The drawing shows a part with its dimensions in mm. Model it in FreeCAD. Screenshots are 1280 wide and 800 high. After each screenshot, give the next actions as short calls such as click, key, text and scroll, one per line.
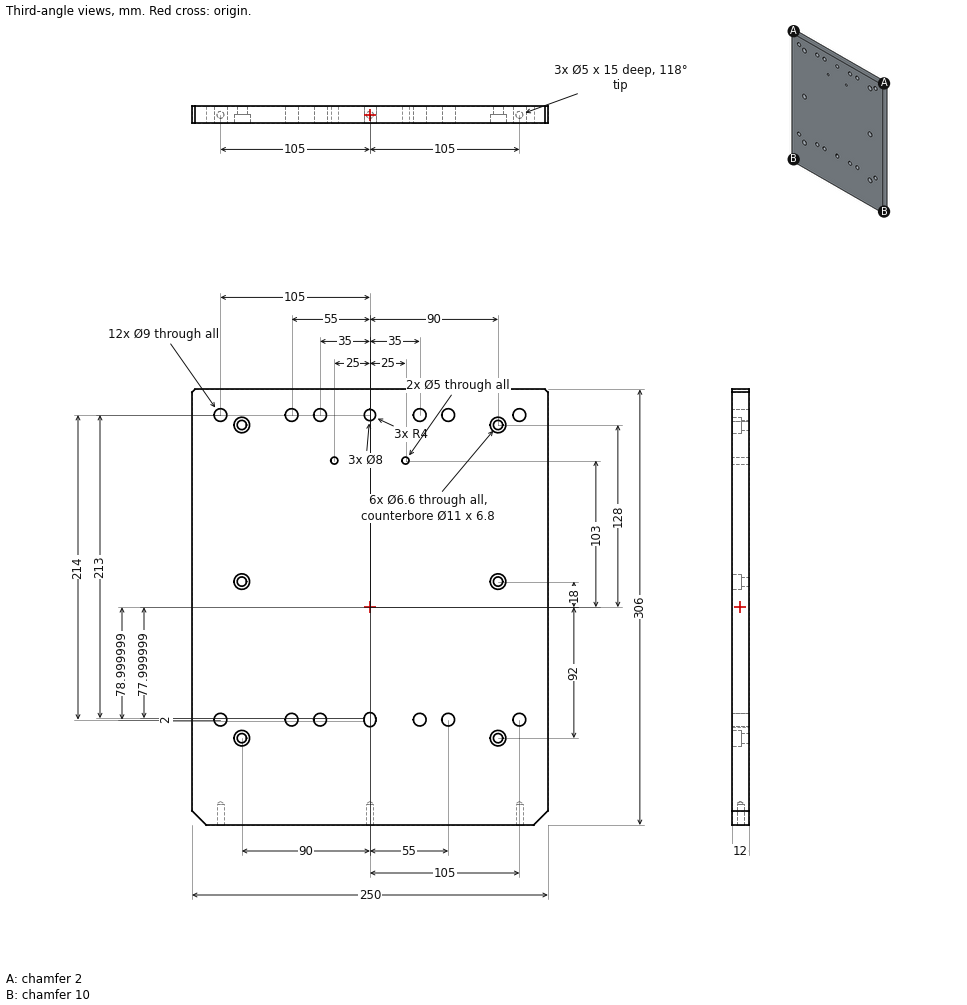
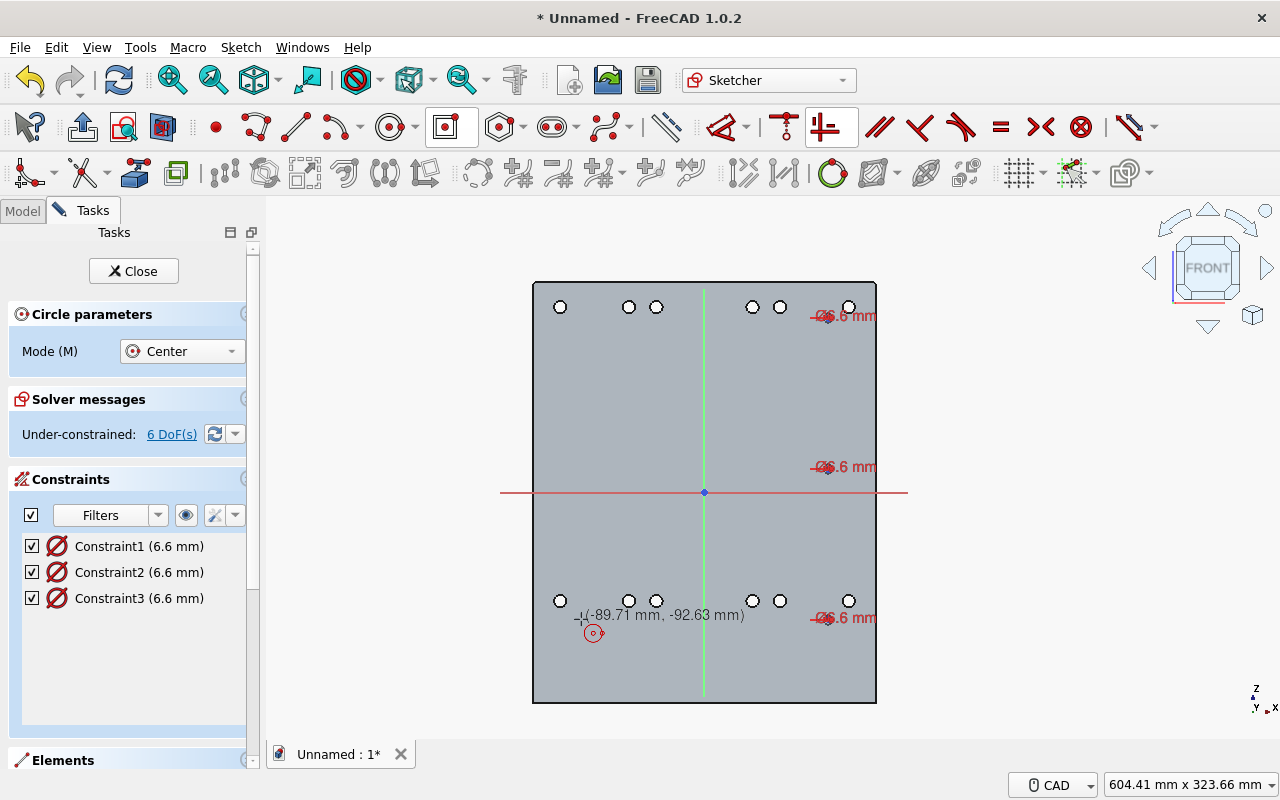
click(581, 619)
move(584, 616)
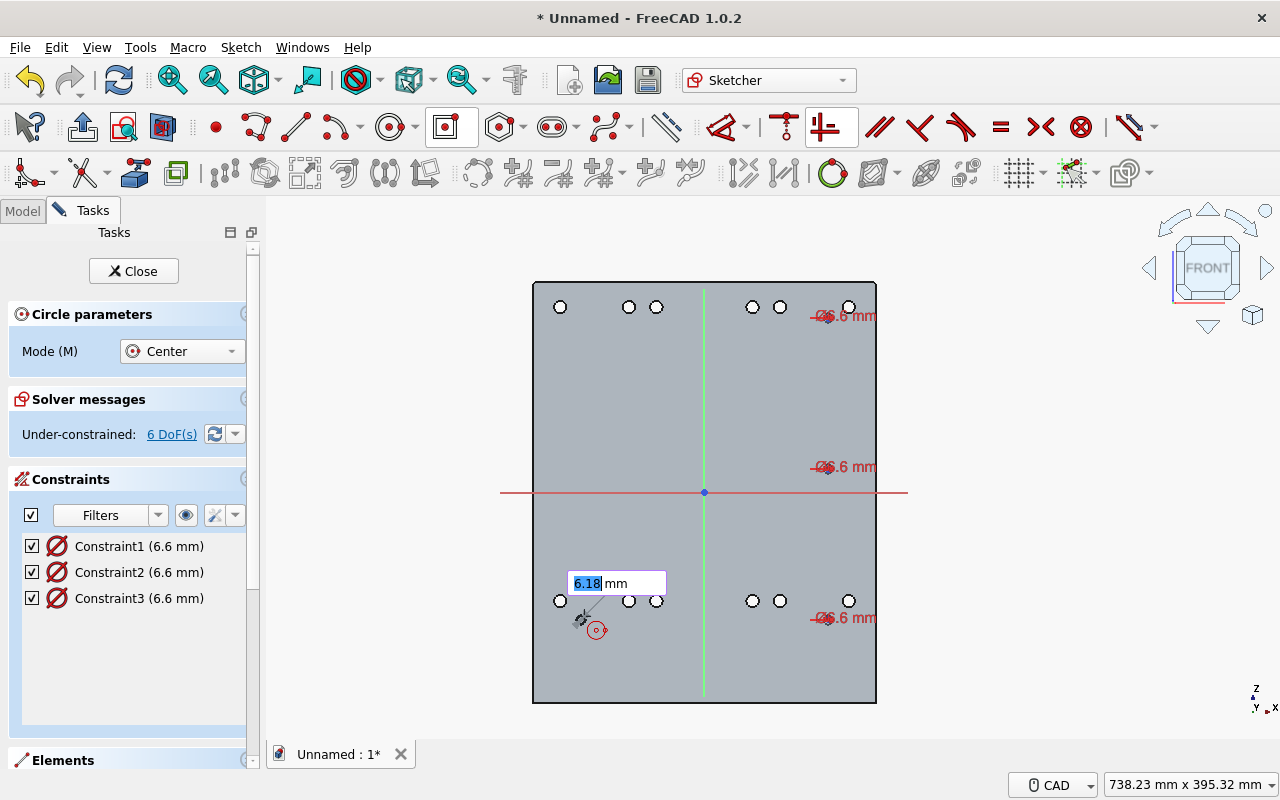
text(6.6)
key(Return)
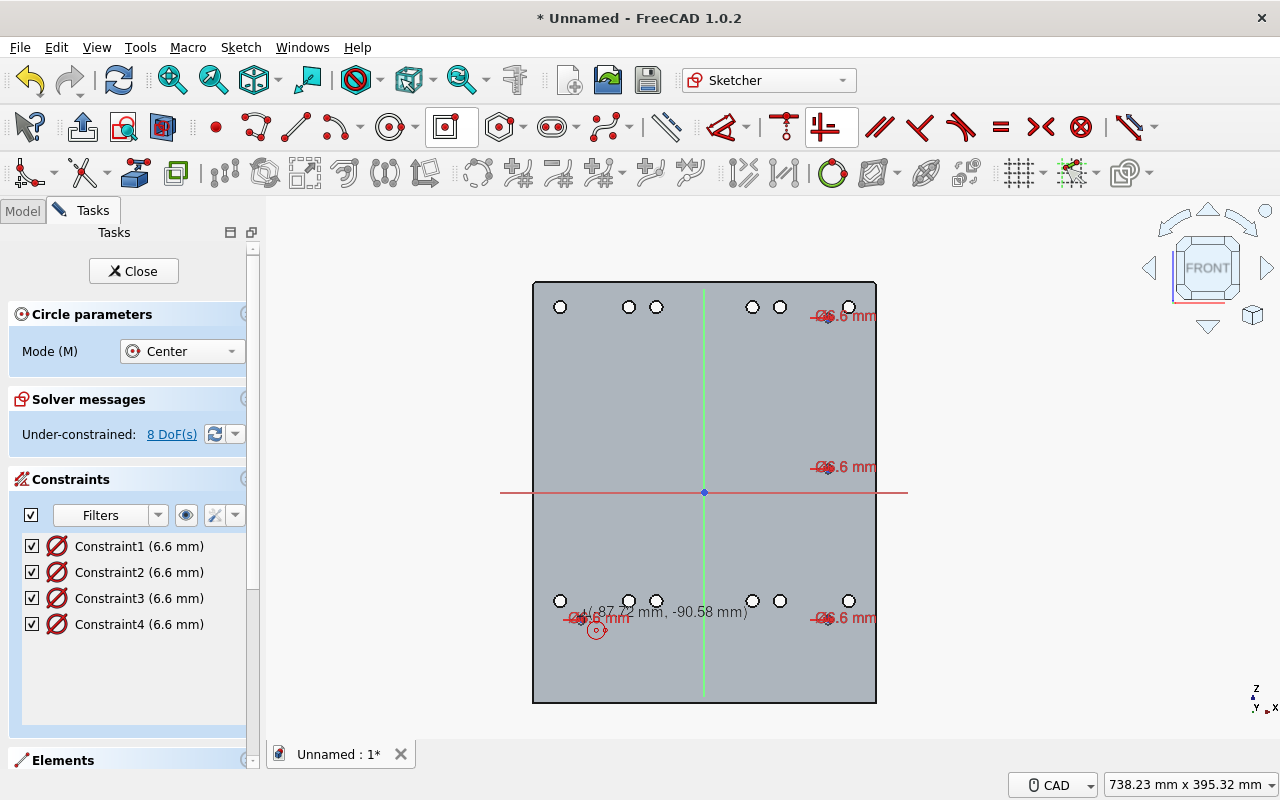
scroll(581, 468, up, 9)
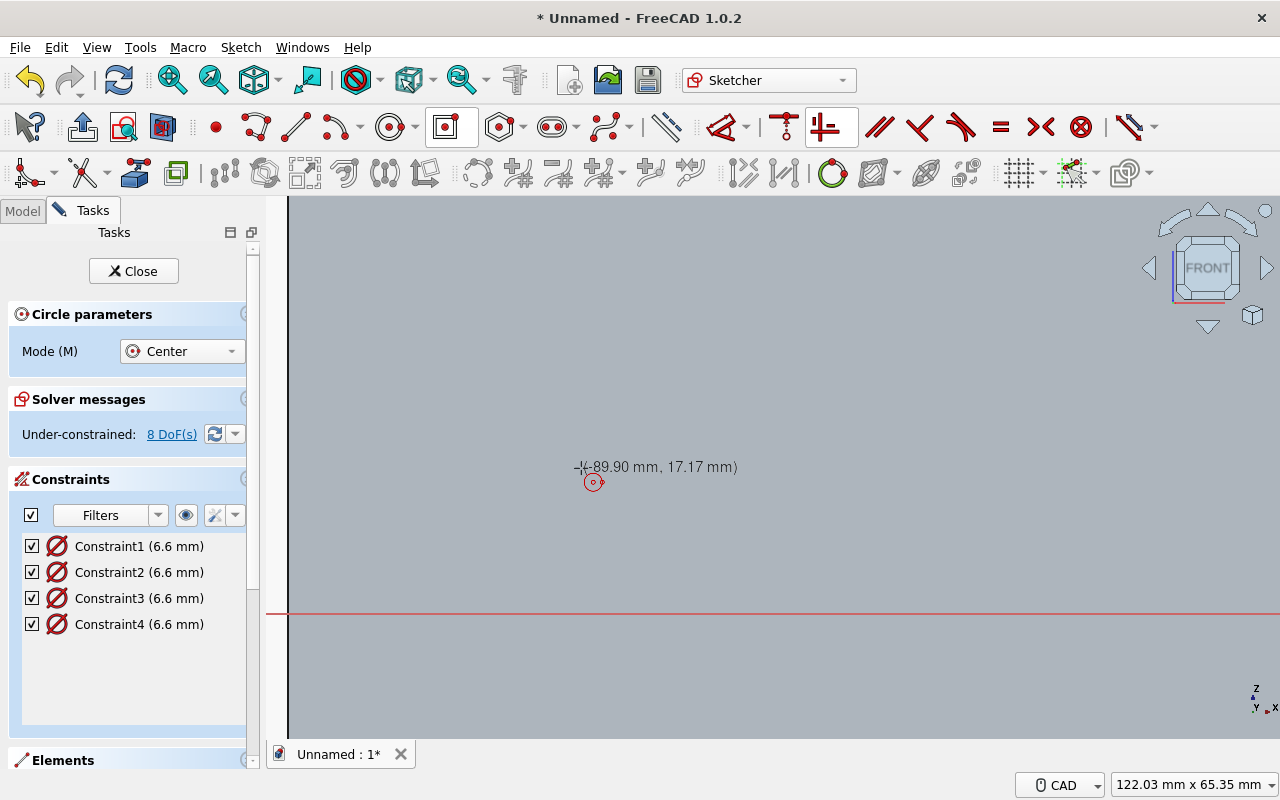
scroll(581, 468, down, 9)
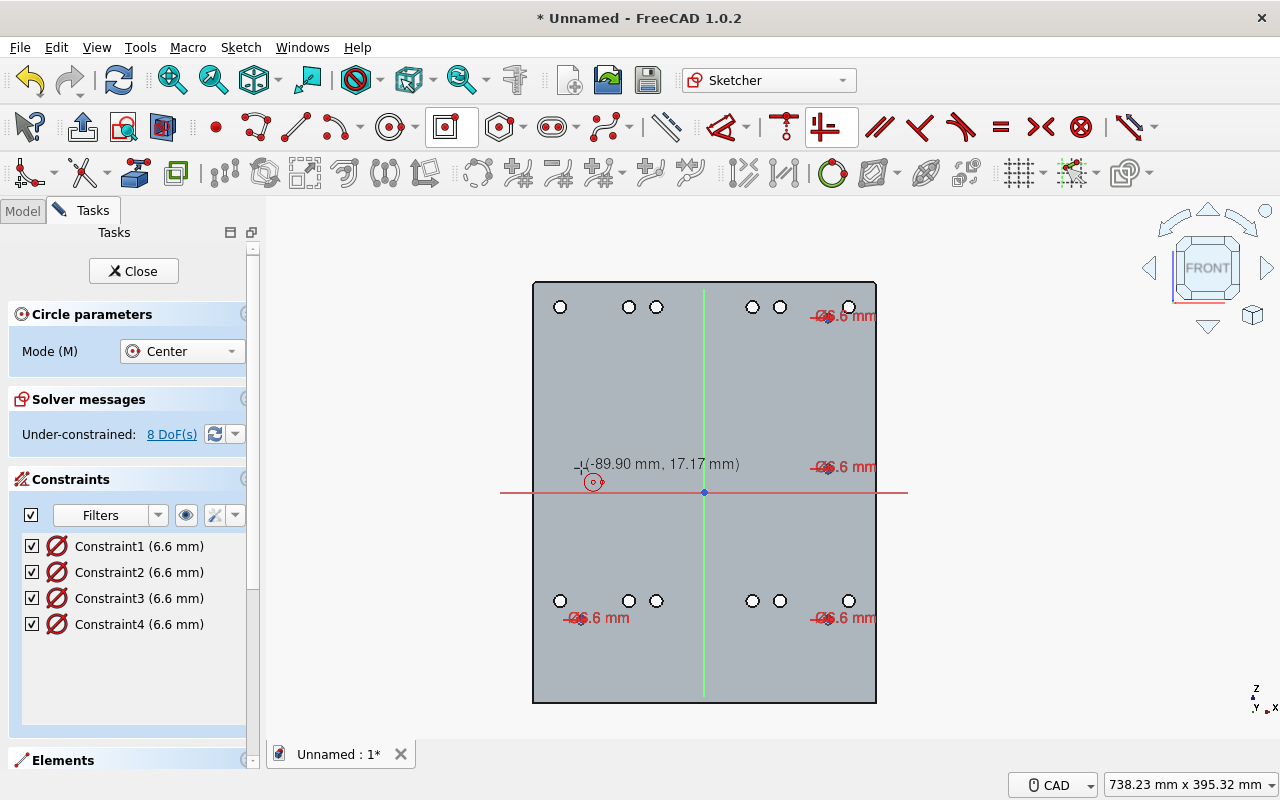
click(581, 468)
move(584, 465)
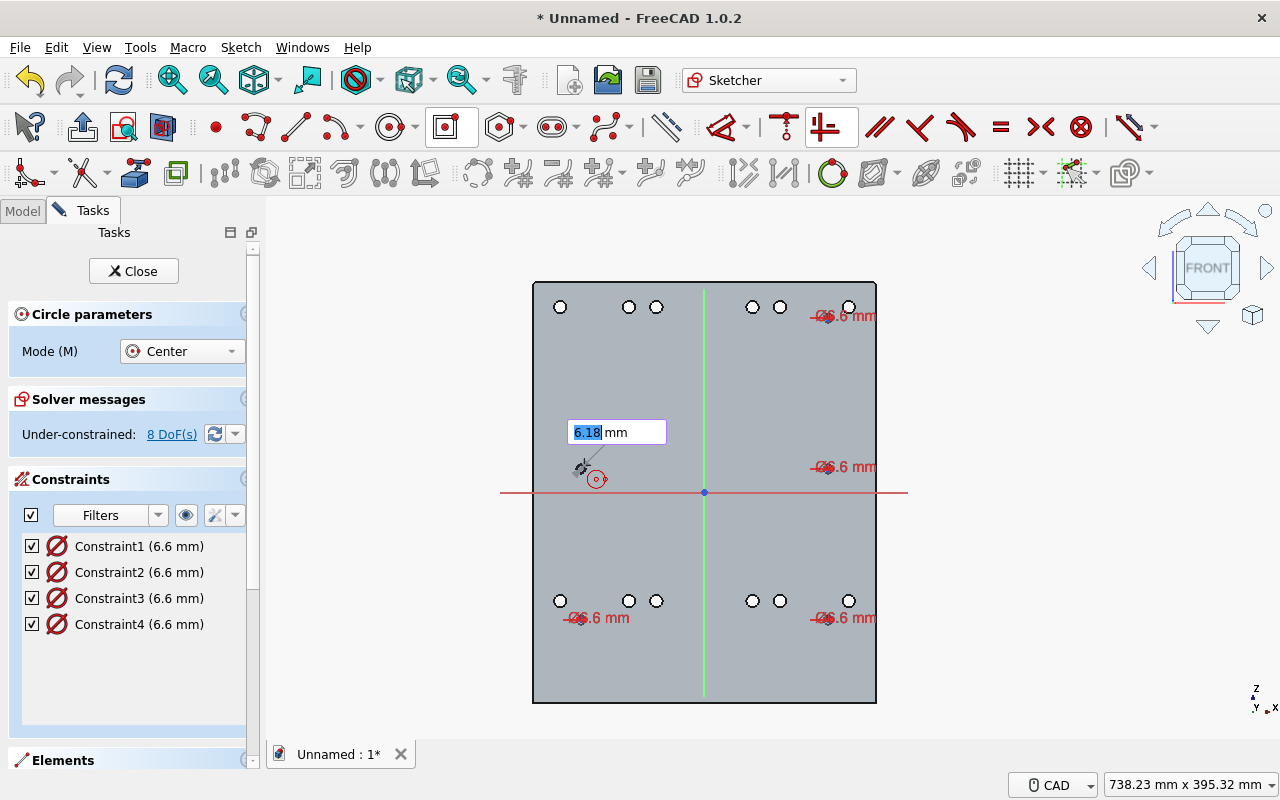
text(6.6)
key(Return)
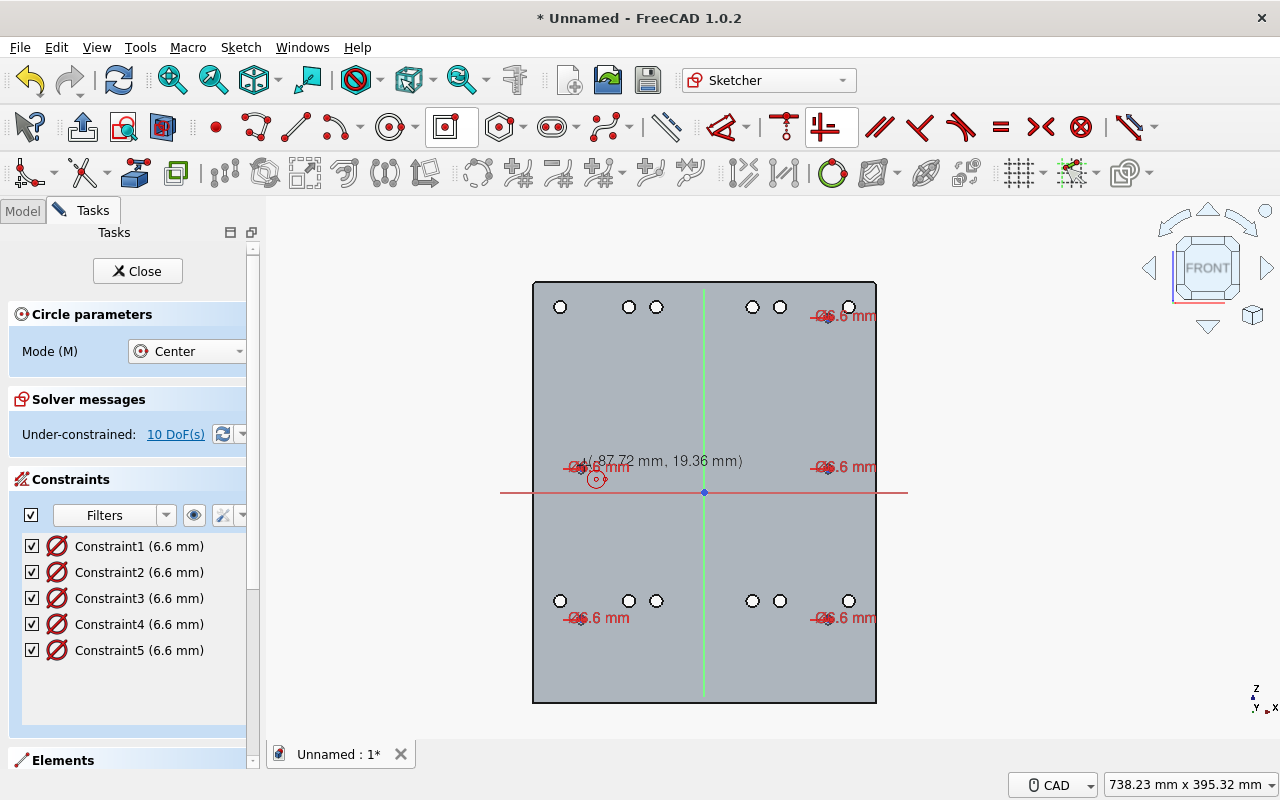
scroll(581, 317, up, 9)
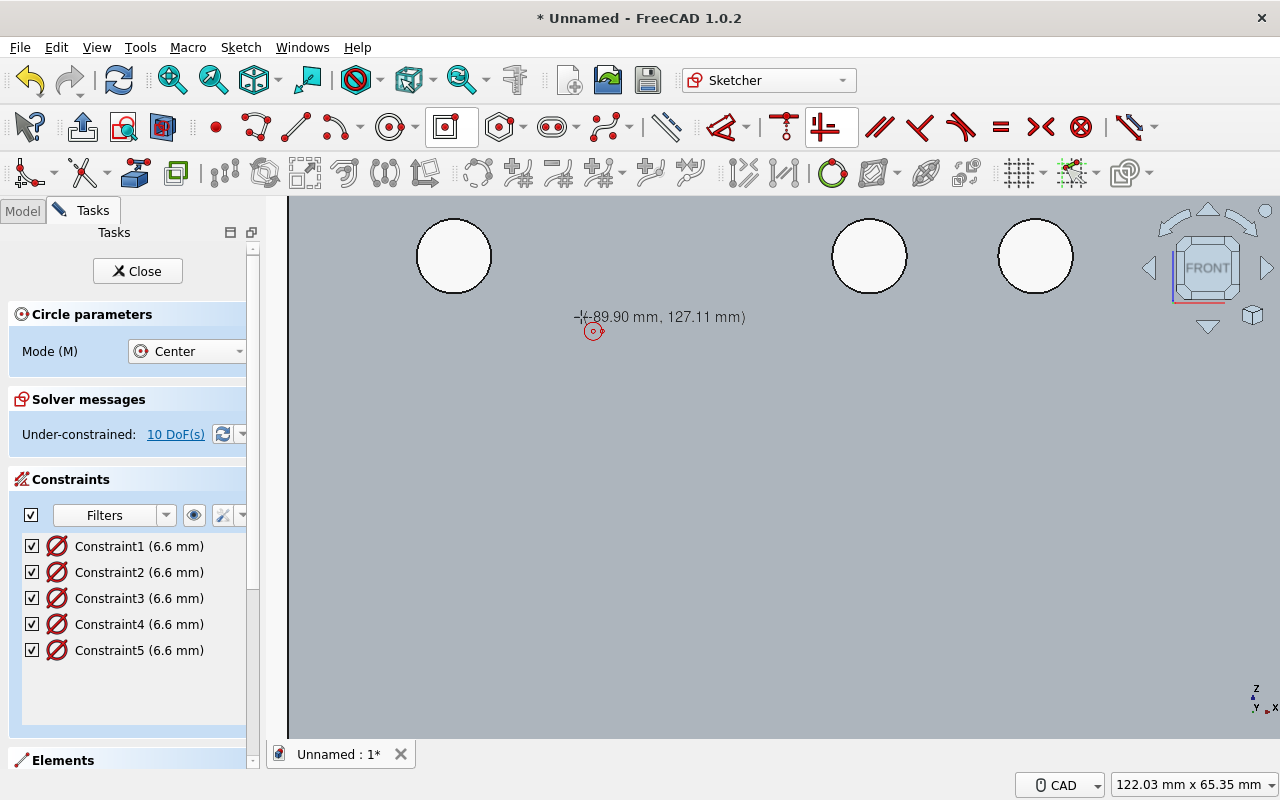
scroll(581, 317, down, 9)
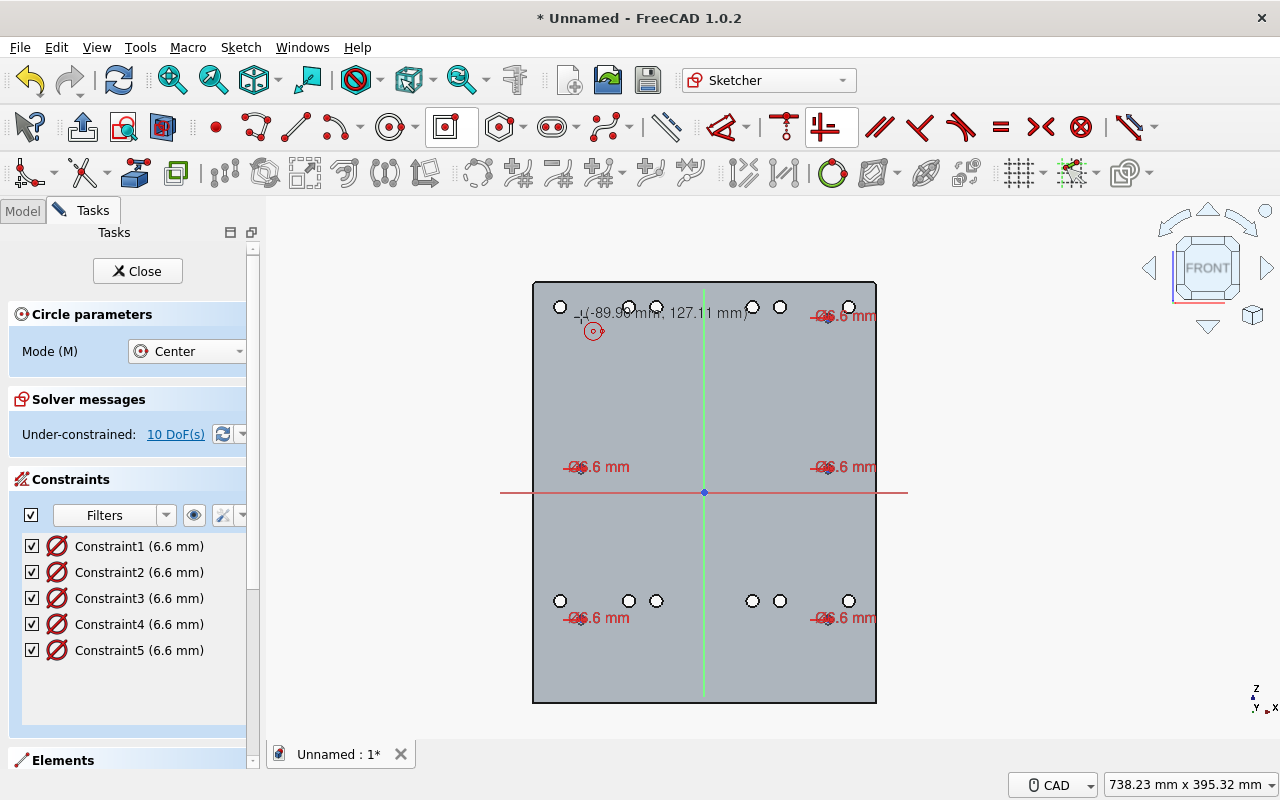
click(581, 317)
move(584, 314)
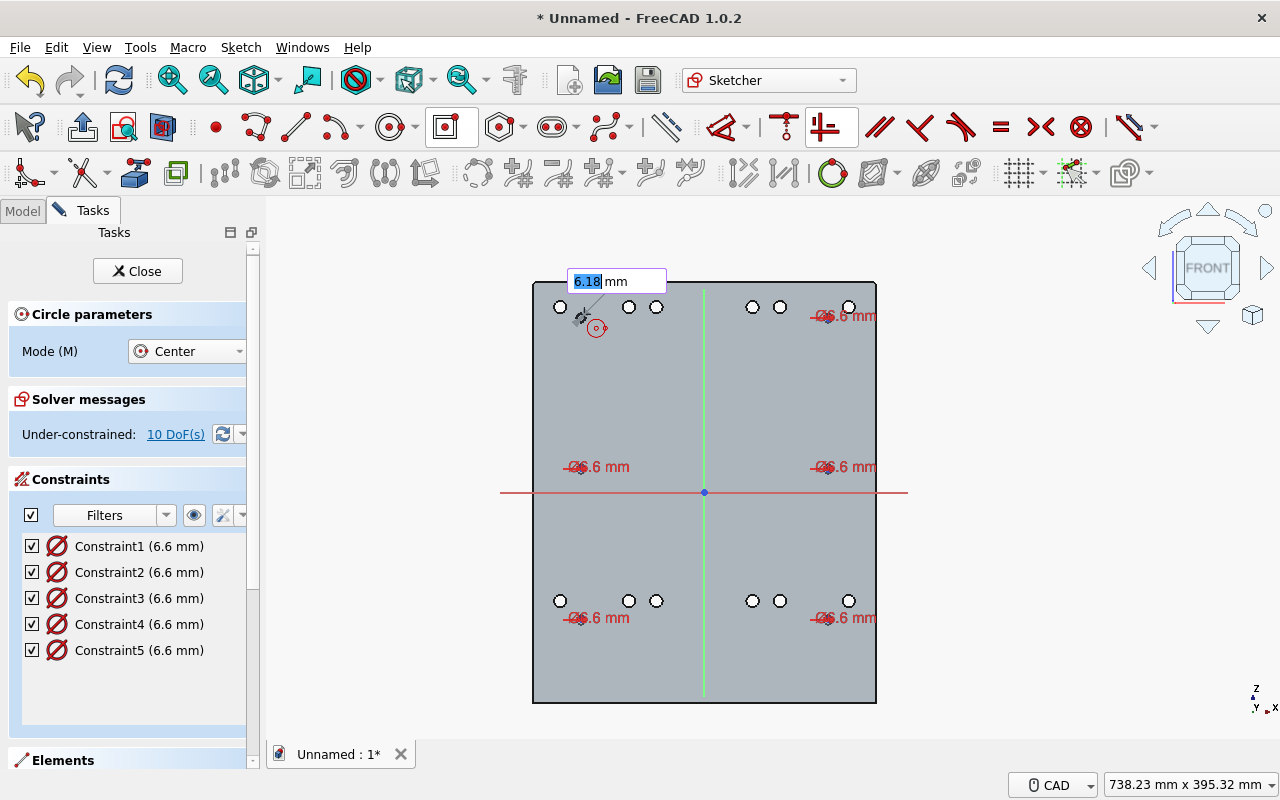
text(6.6)
key(Return)
key(Escape)